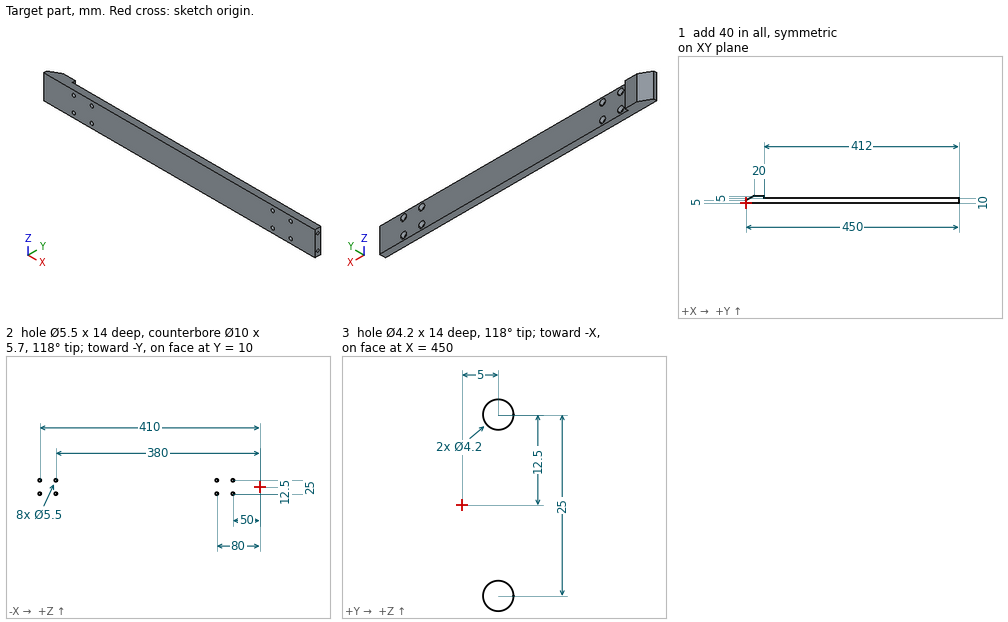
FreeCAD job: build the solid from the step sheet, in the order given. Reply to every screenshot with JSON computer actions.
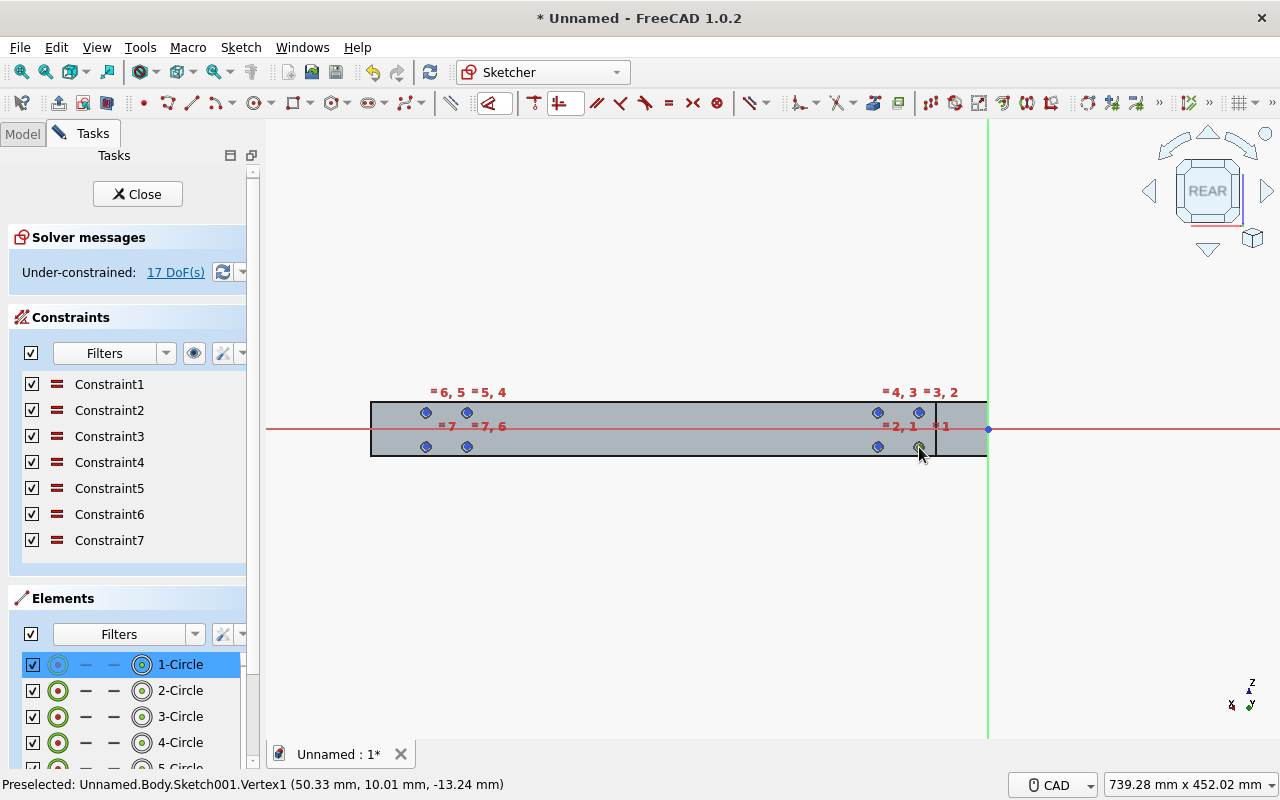
{"action": "left_click", "coordinate": [878, 447]}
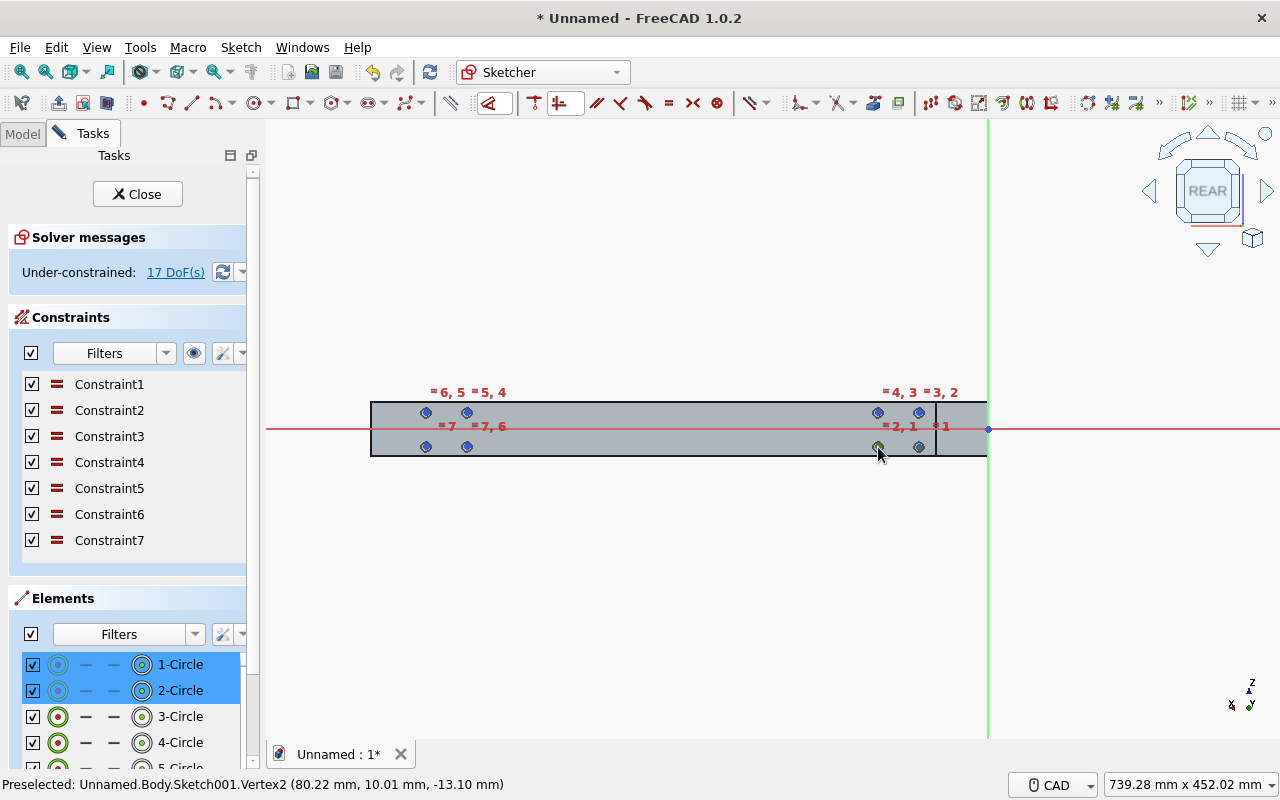
{"action": "left_click", "coordinate": [578, 104]}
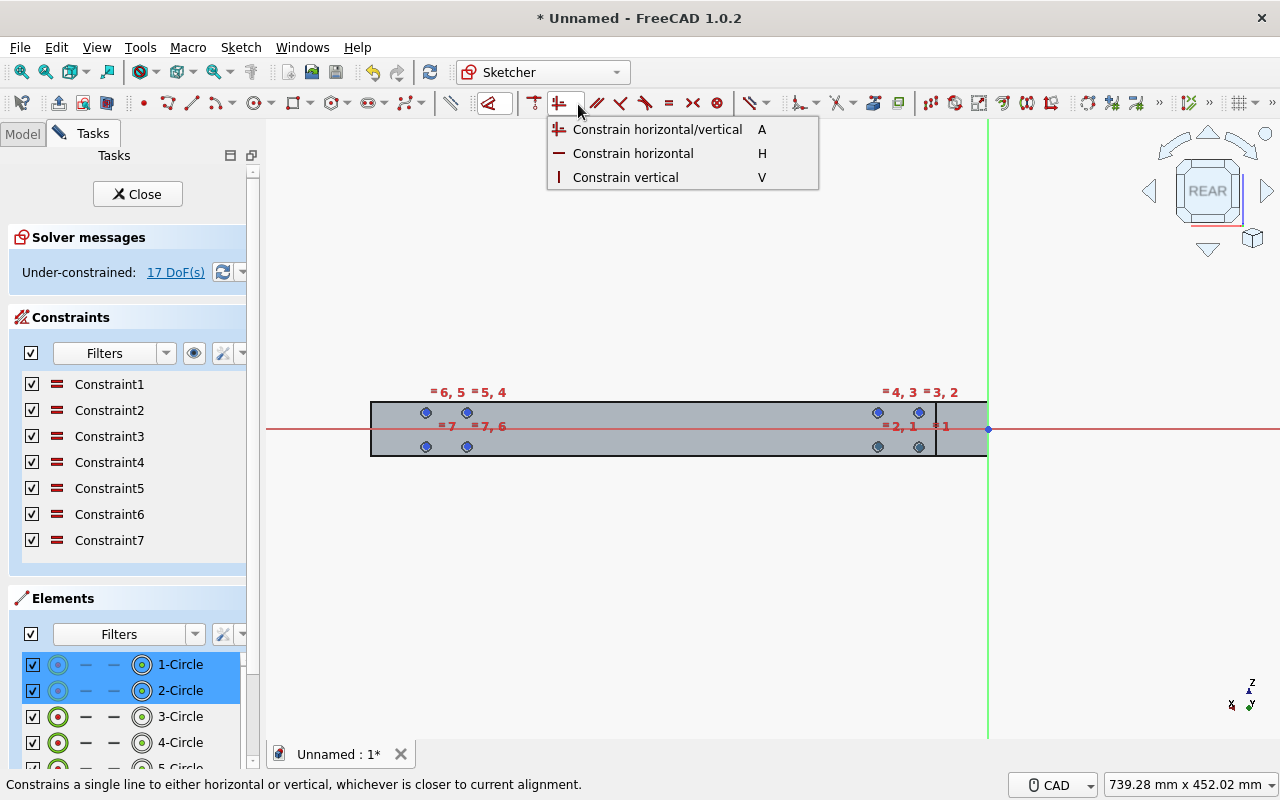
{"action": "left_click", "coordinate": [683, 153]}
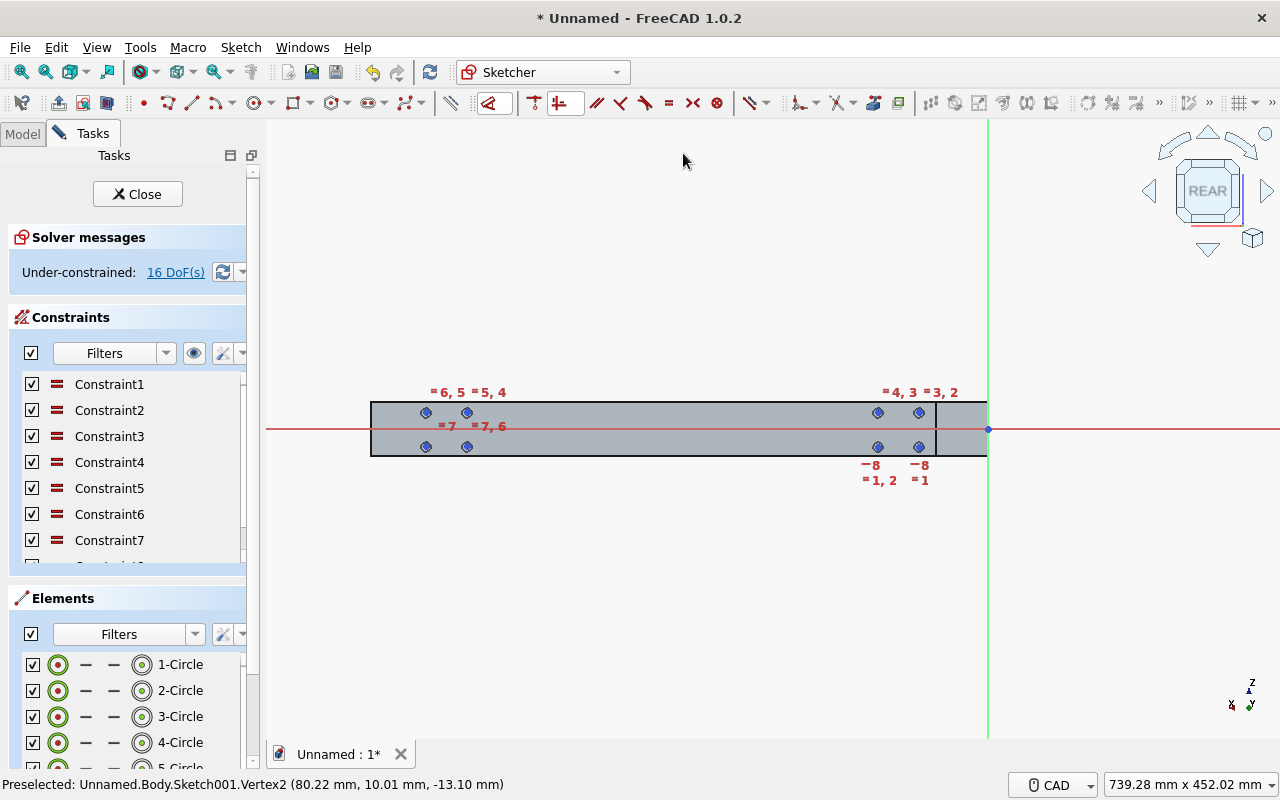
{"action": "left_click", "coordinate": [919, 447]}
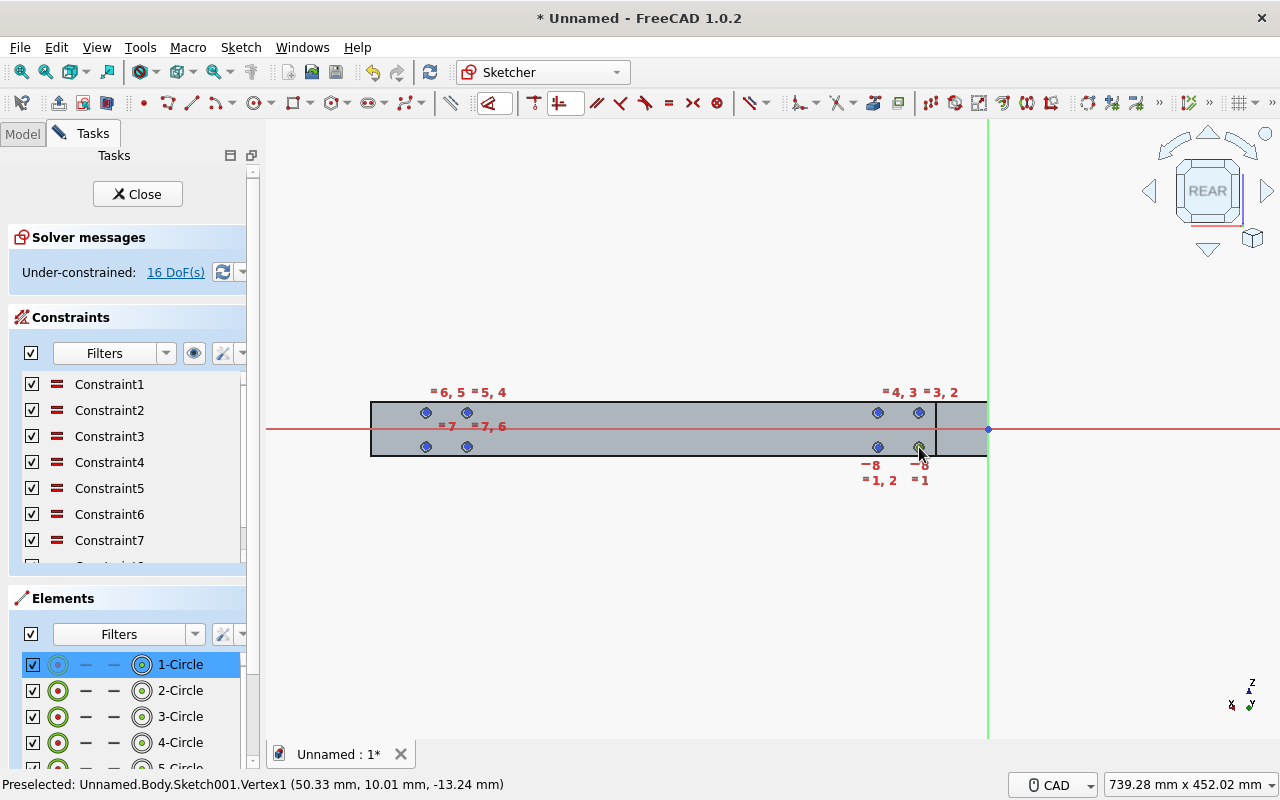
{"action": "left_click", "coordinate": [919, 413]}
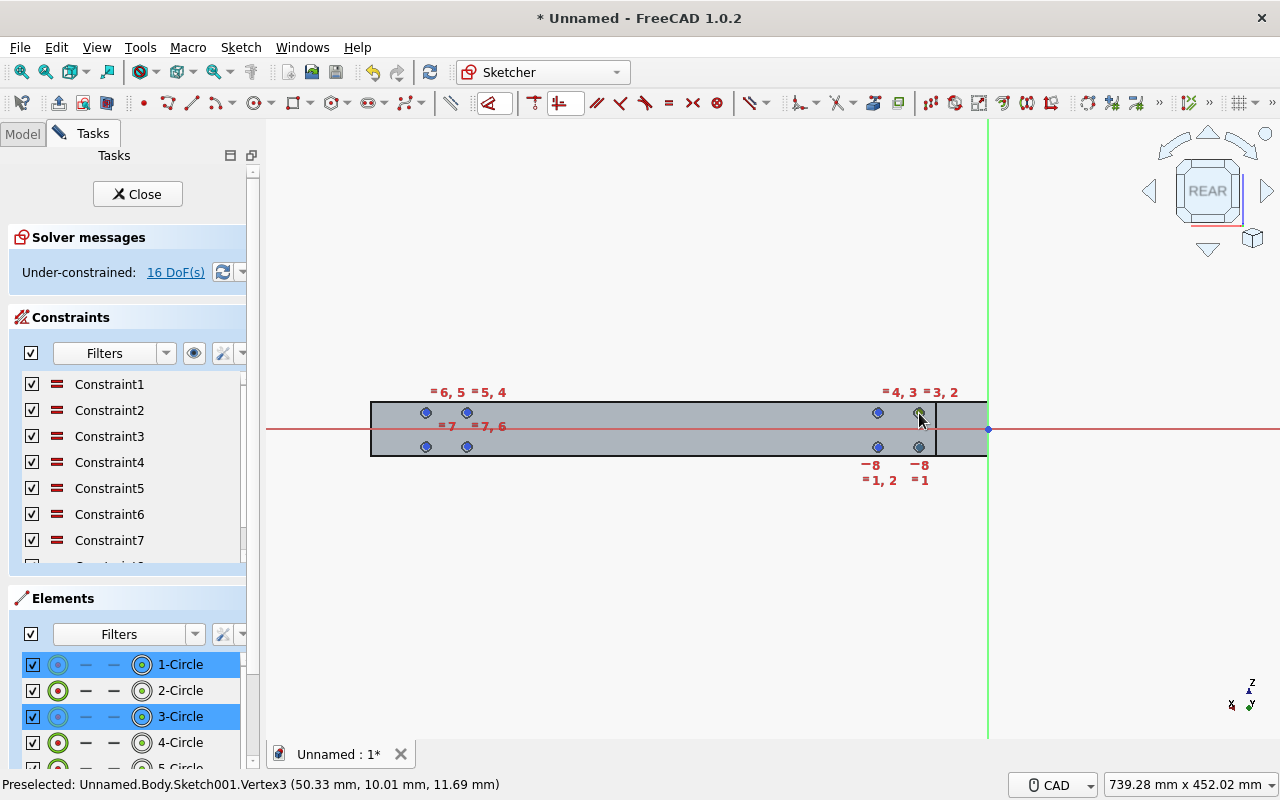
{"action": "key", "text": "v"}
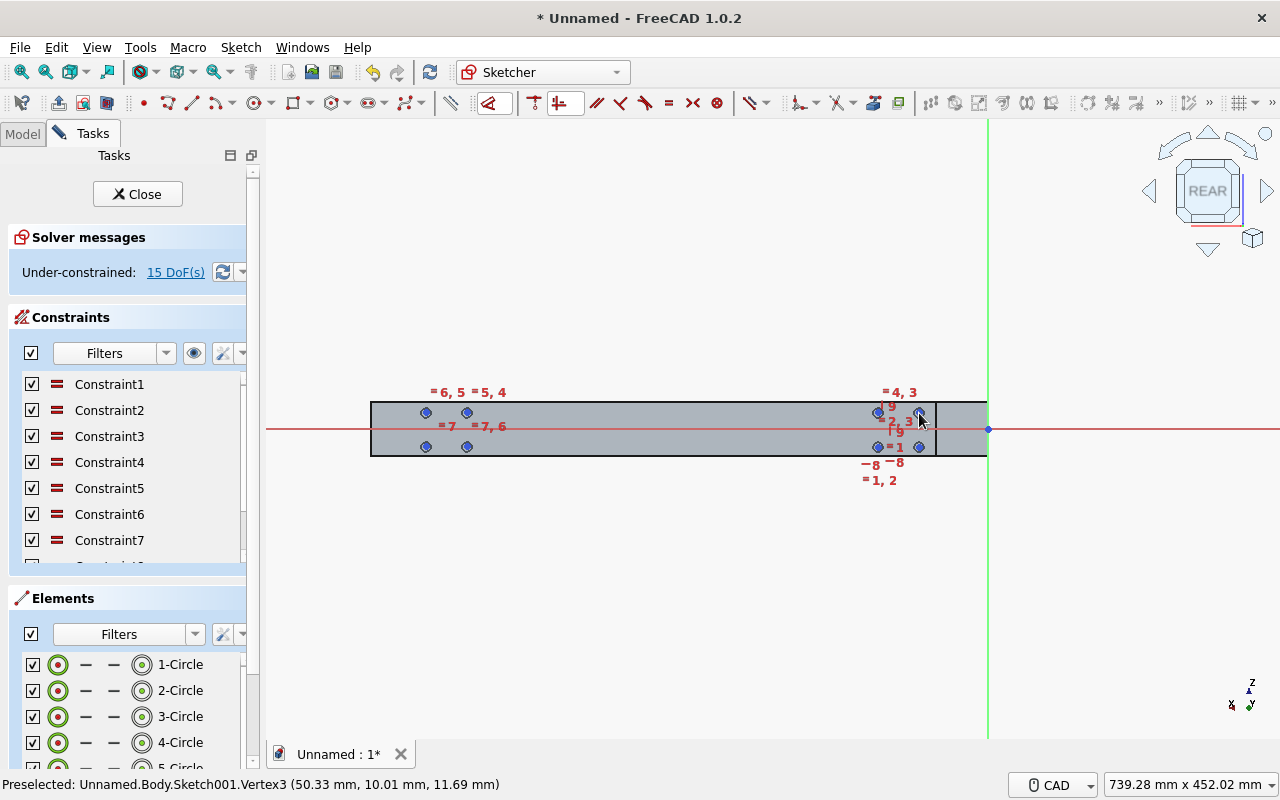
{"action": "left_click", "coordinate": [878, 447]}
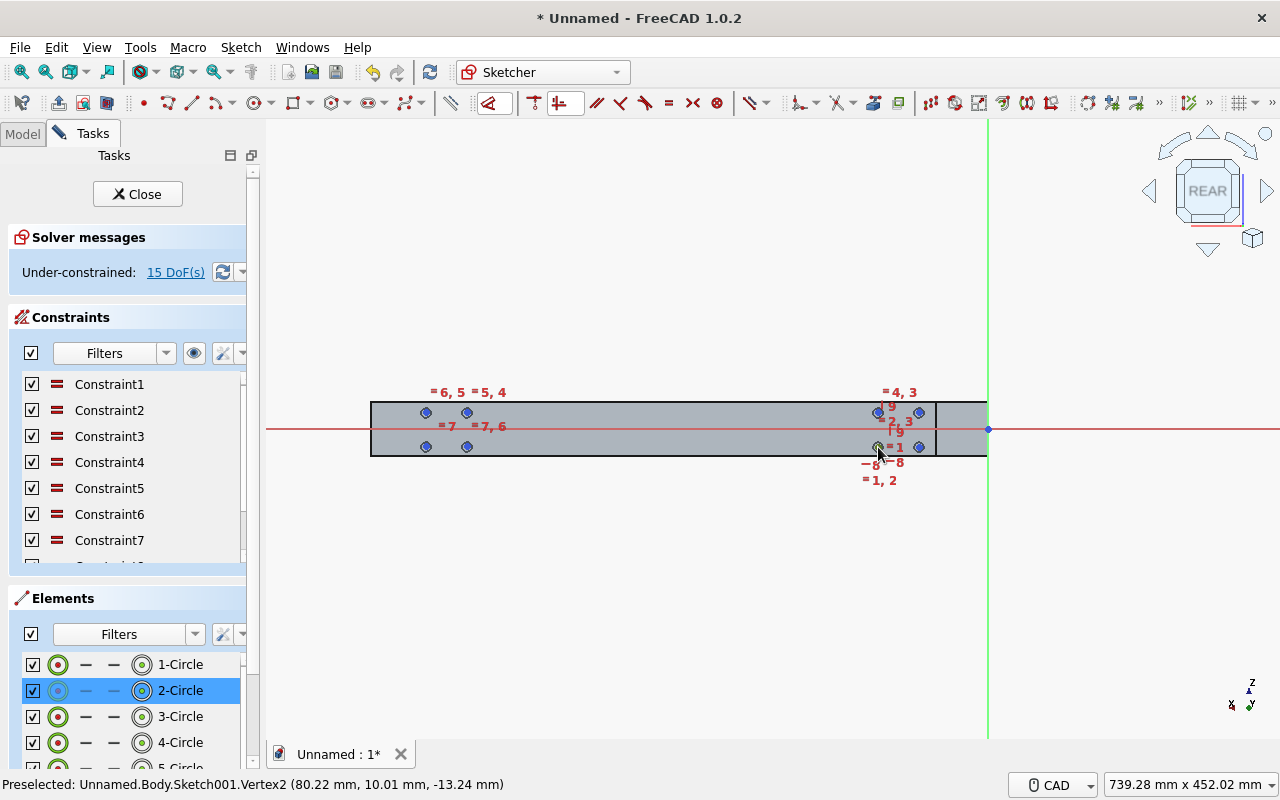
{"action": "scroll", "coordinate": [878, 413], "scroll_direction": "up", "scroll_amount": 4}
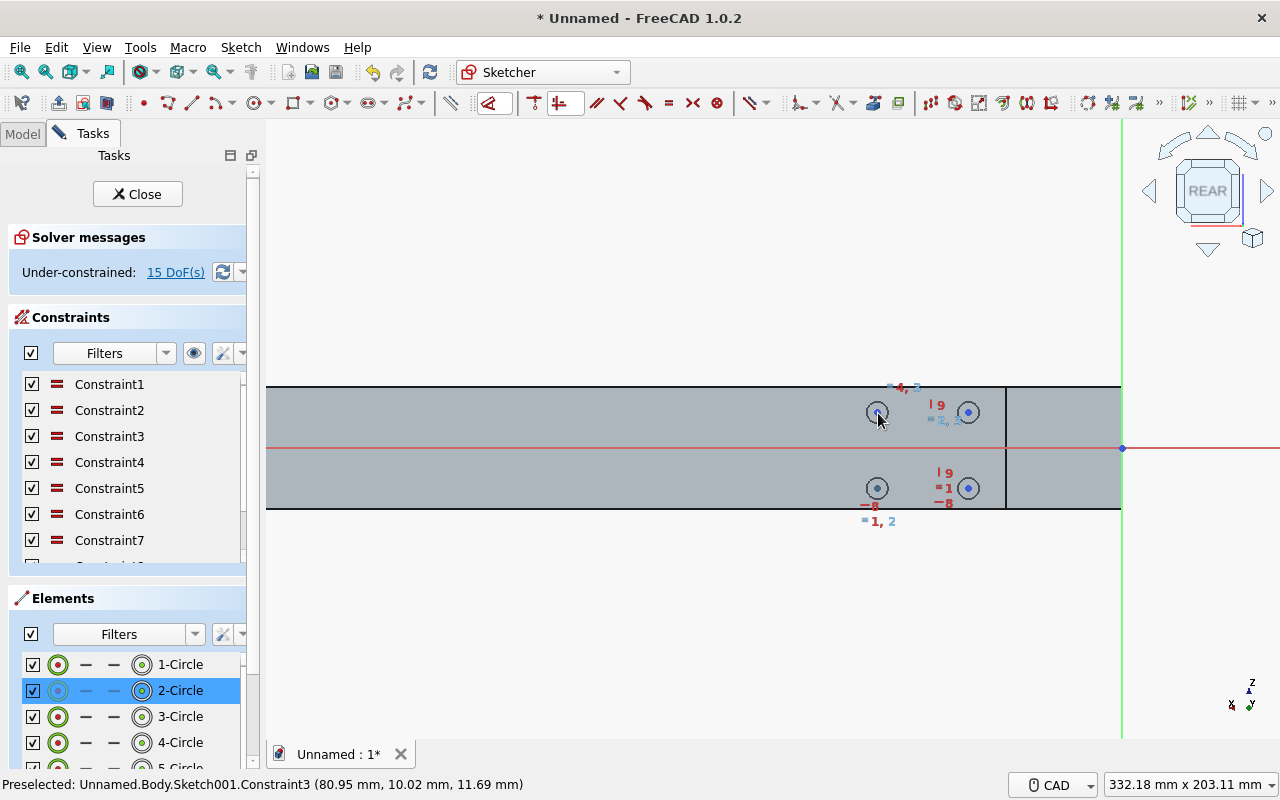
{"action": "left_click", "coordinate": [877, 412]}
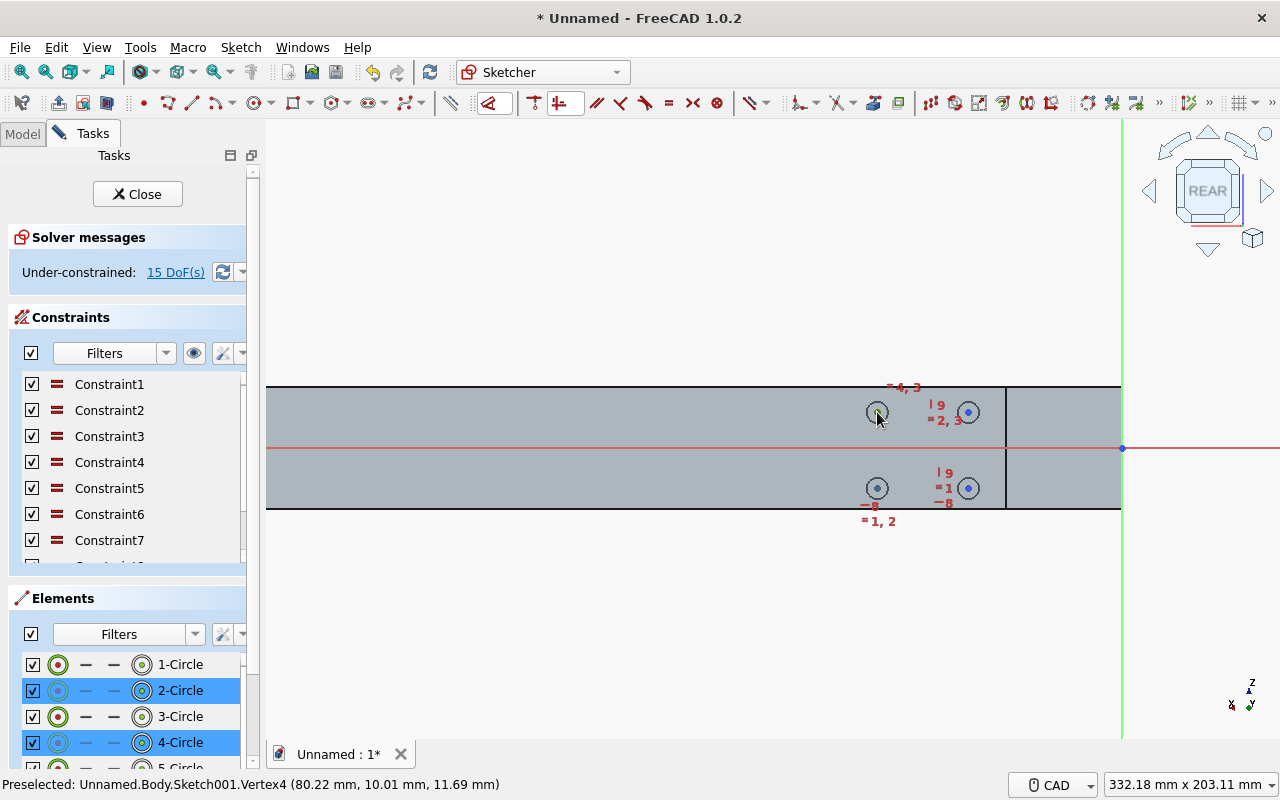
{"action": "left_click", "coordinate": [578, 104]}